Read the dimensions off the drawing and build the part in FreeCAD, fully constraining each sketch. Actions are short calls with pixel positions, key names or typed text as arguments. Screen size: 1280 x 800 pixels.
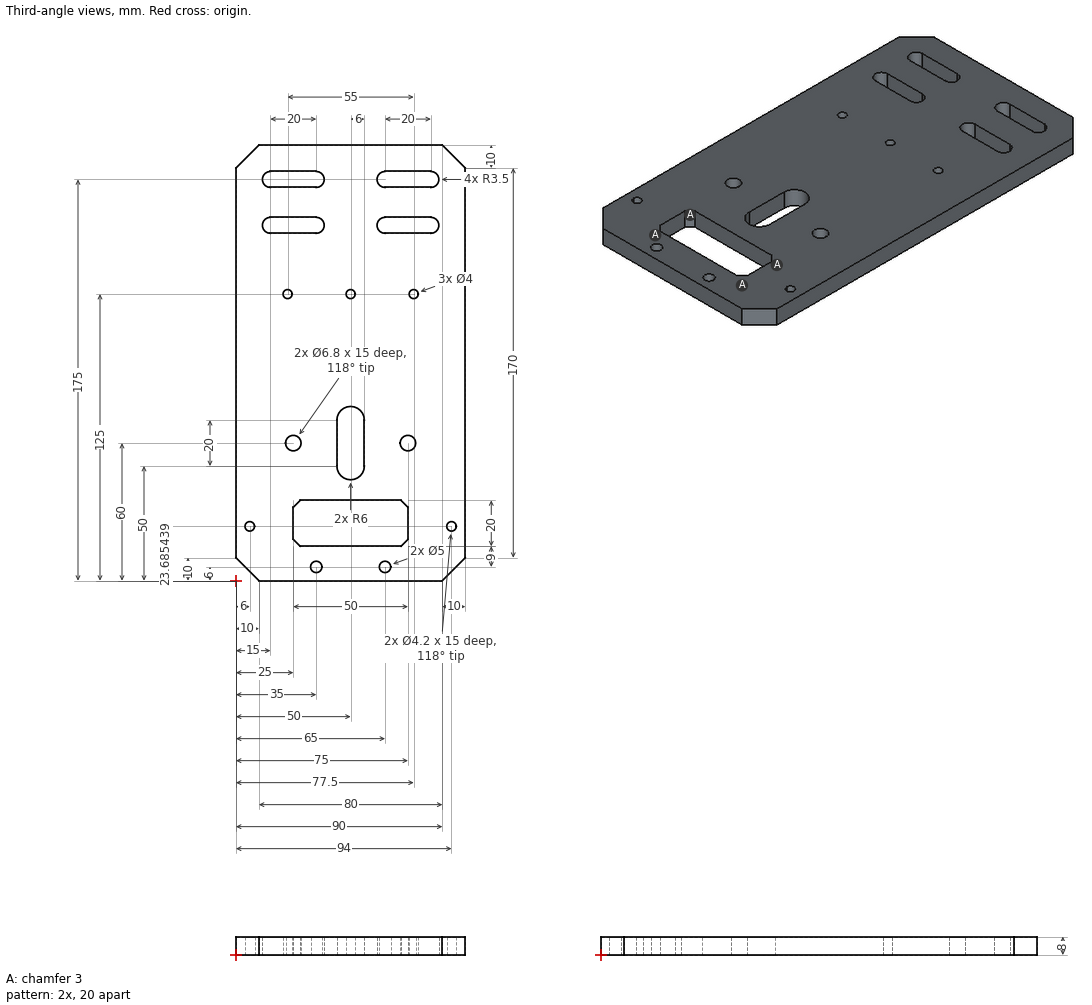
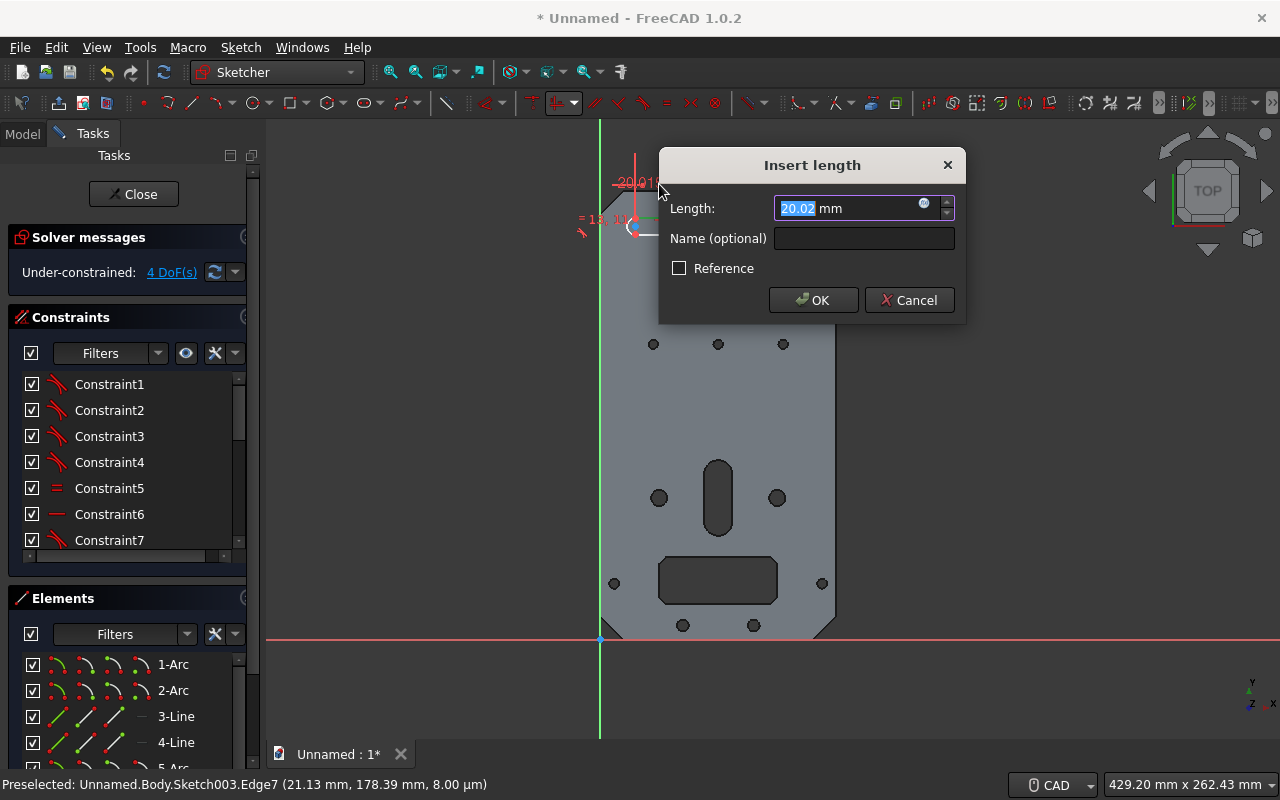
text(20)
key(Return)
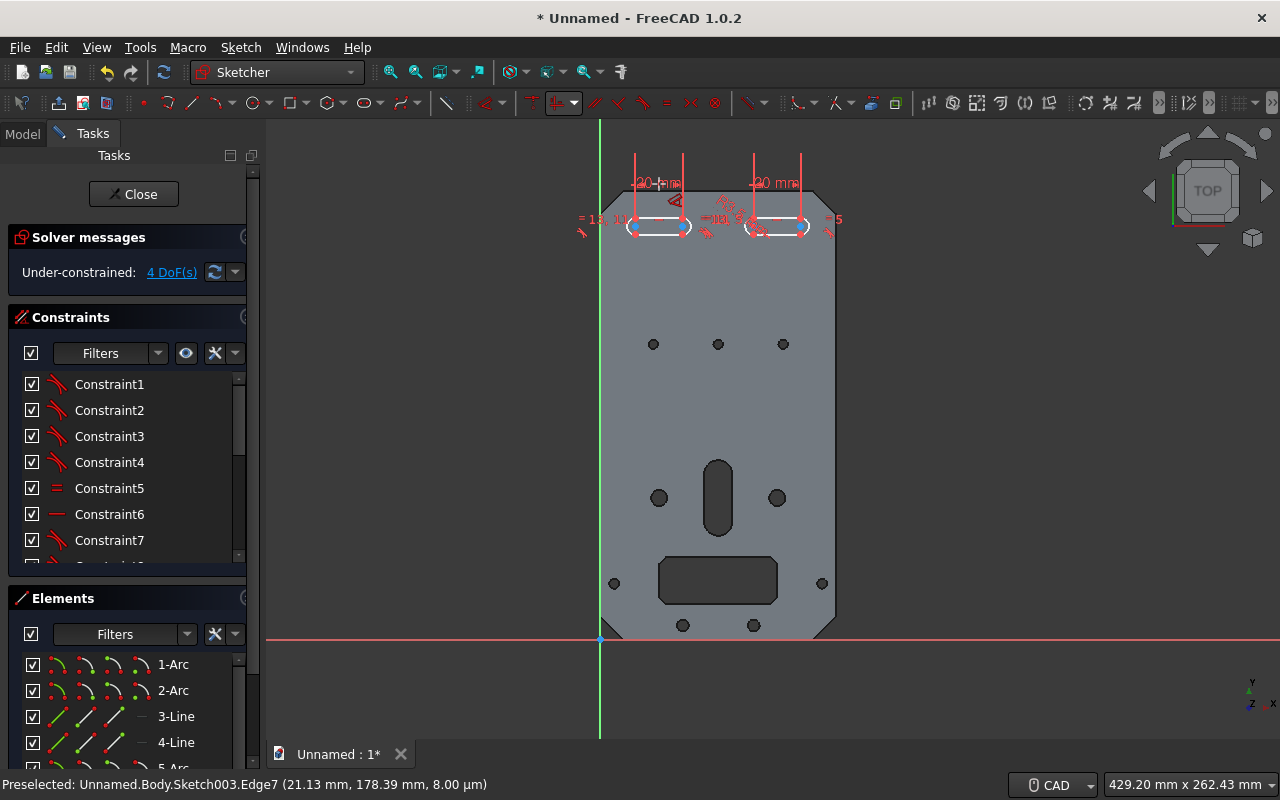
scroll(754, 218, up, 2)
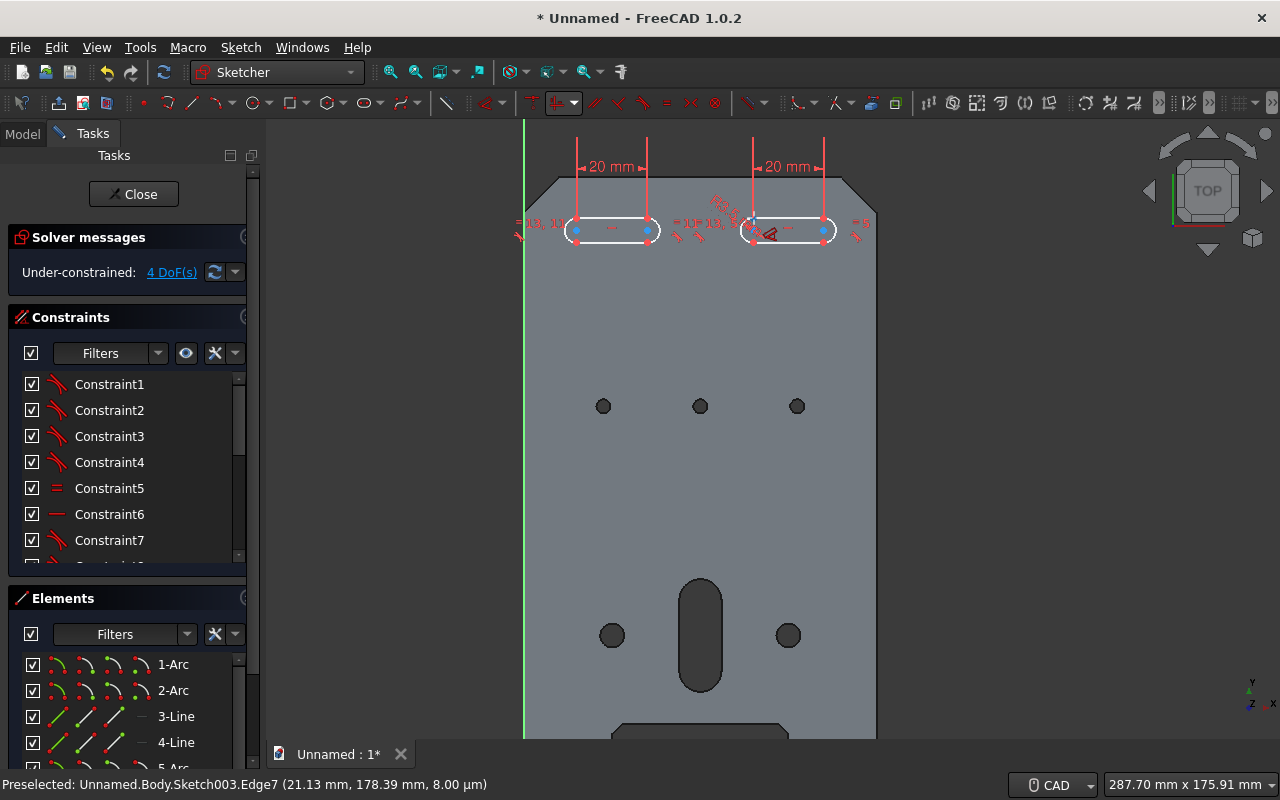
click(753, 218)
click(691, 184)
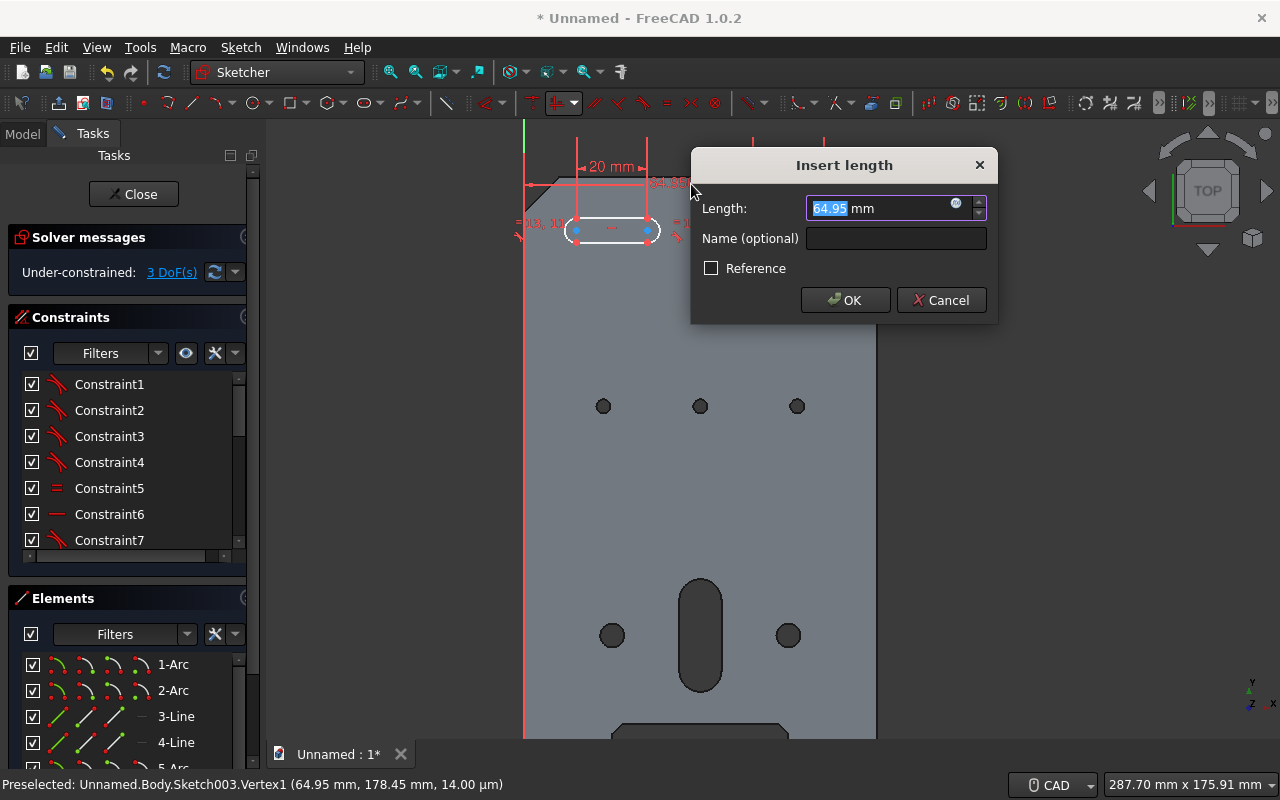
text(65)
key(Return)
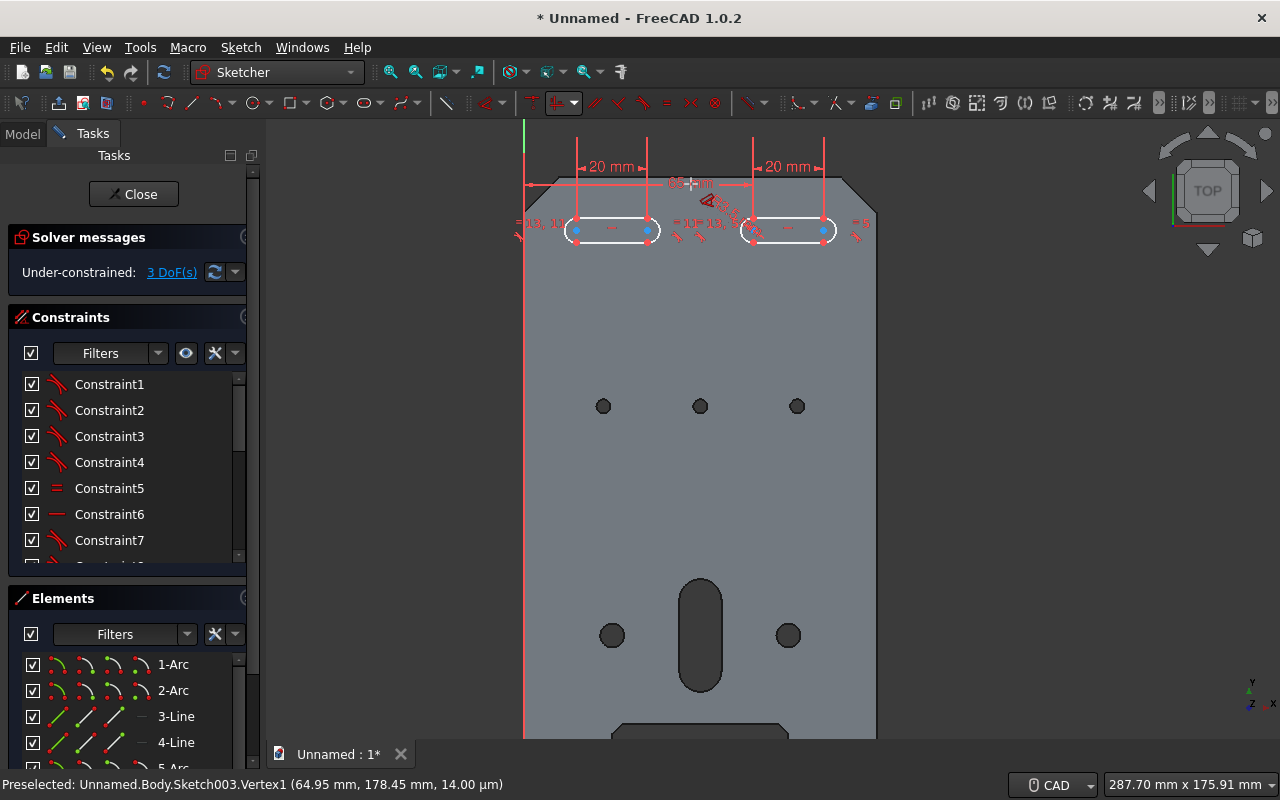
click(577, 218)
click(538, 184)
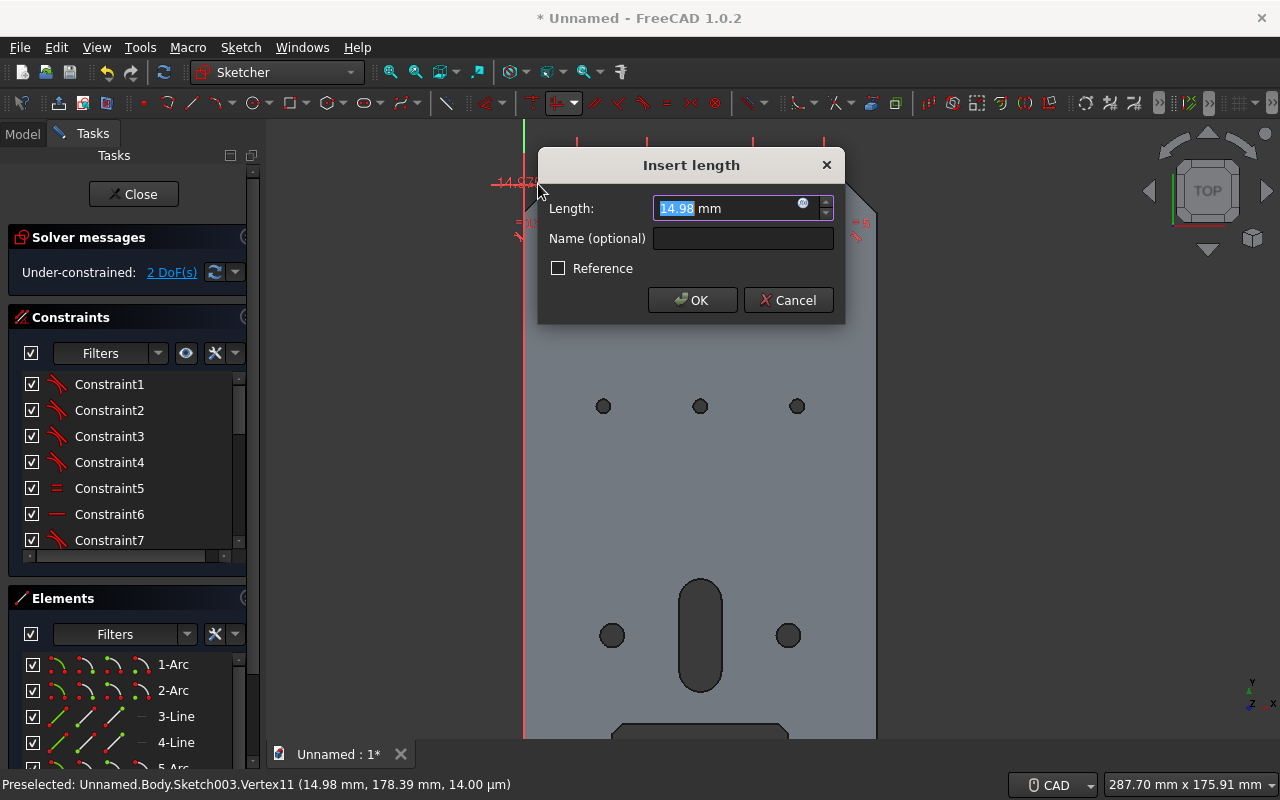
text(15)
key(Return)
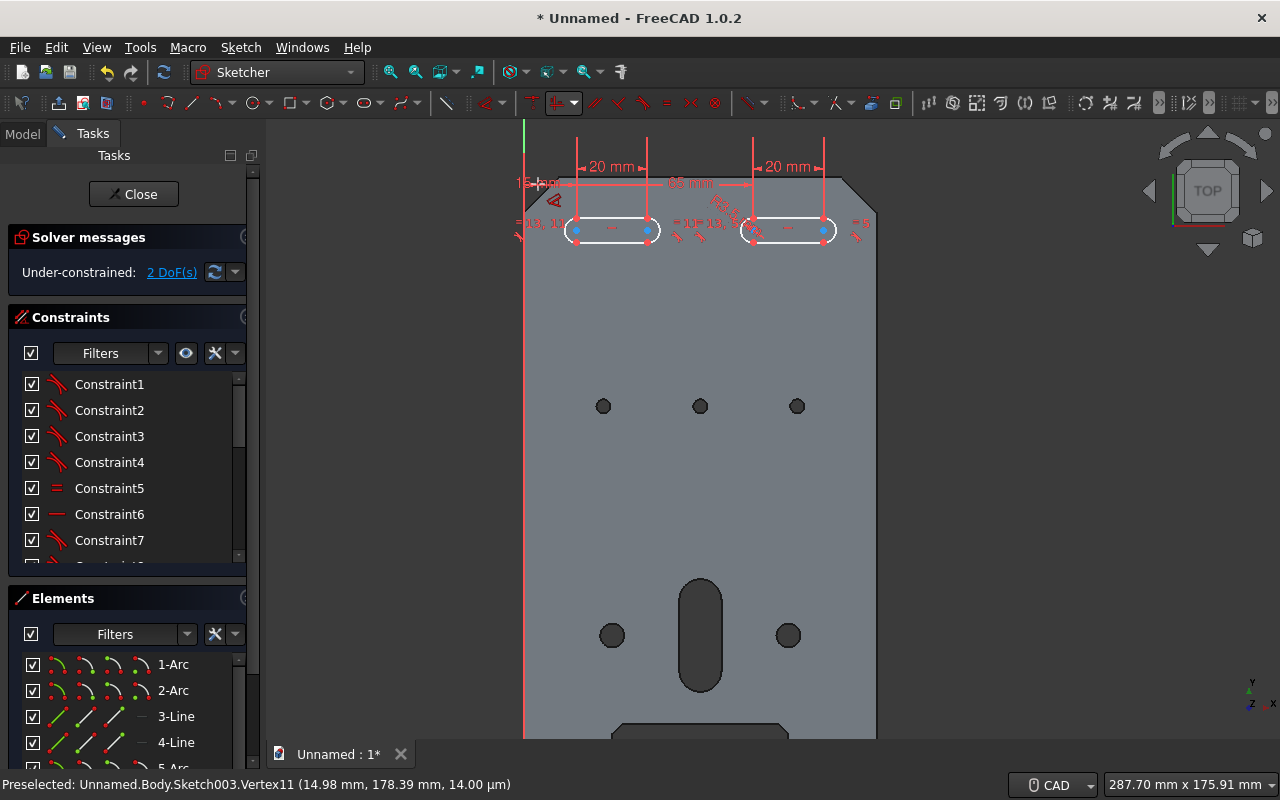
click(753, 230)
click(490, 471)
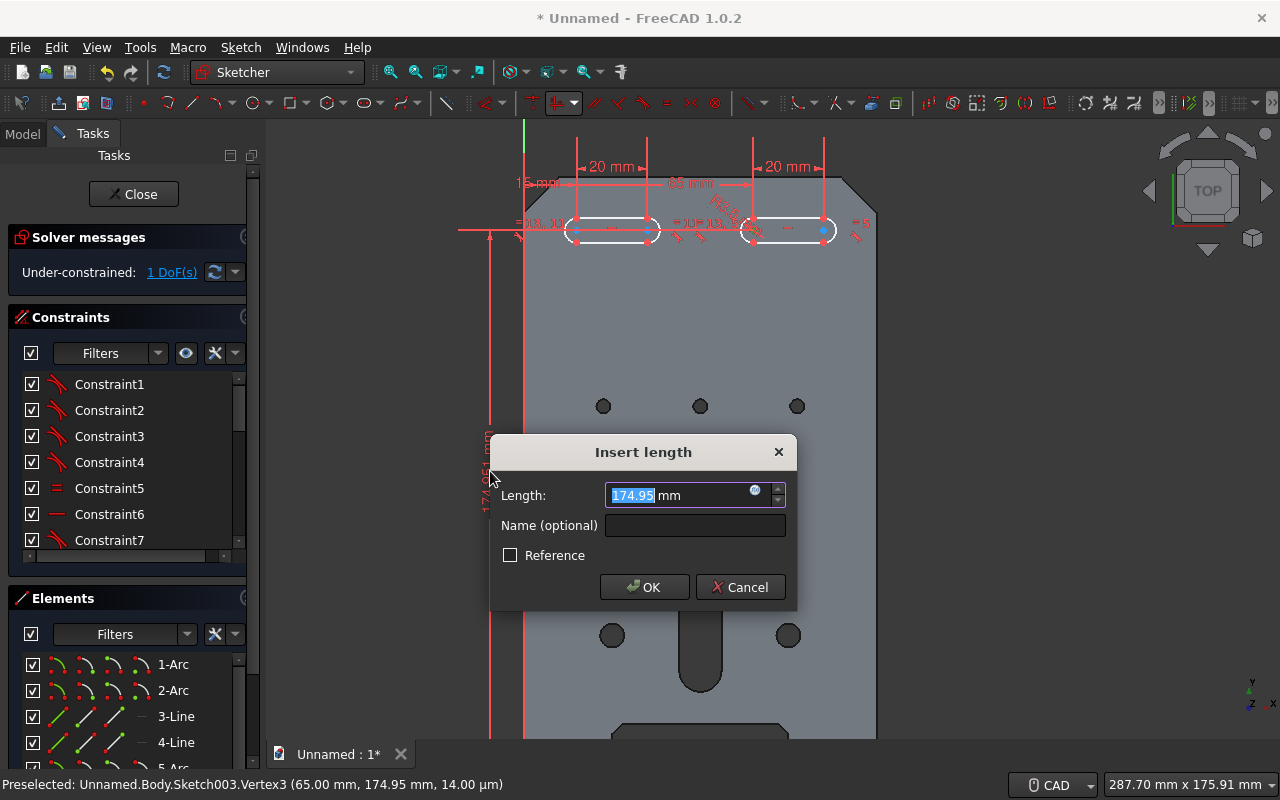
text(175)
key(Return)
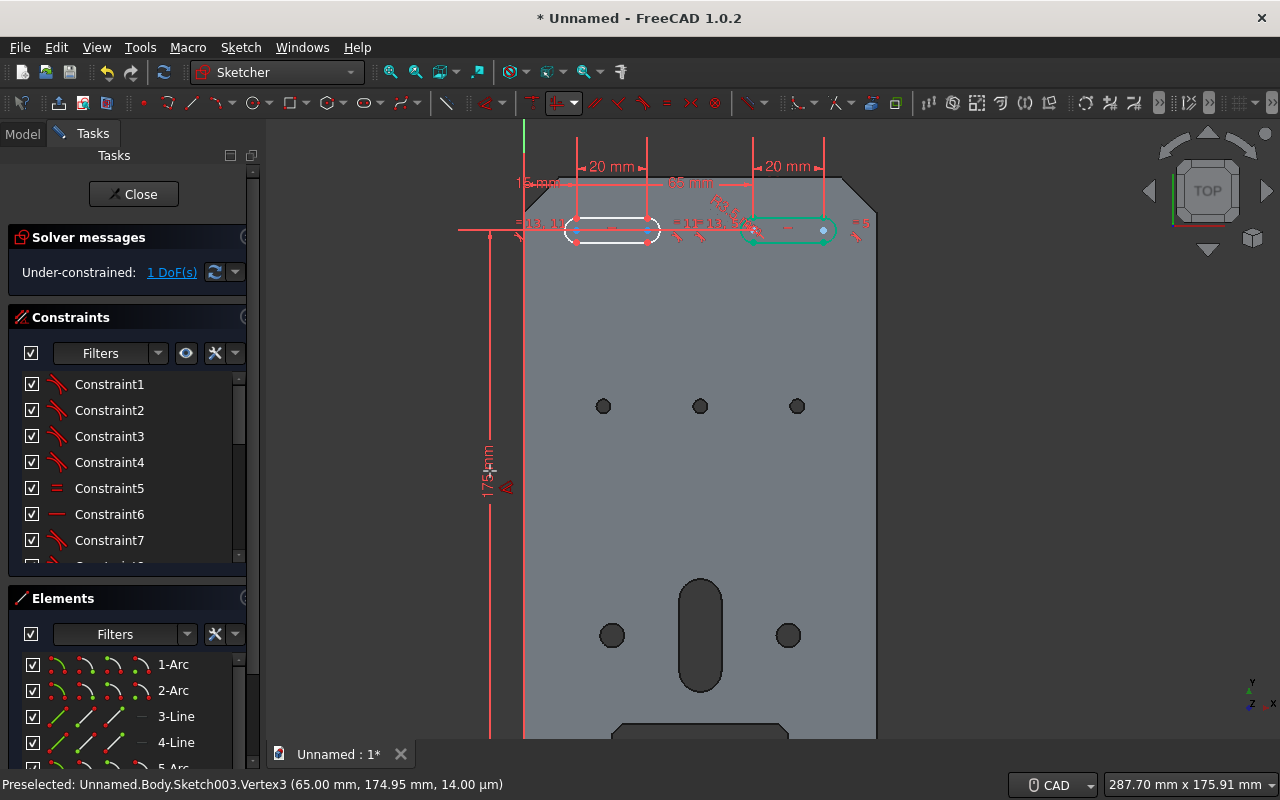
click(577, 231)
click(490, 360)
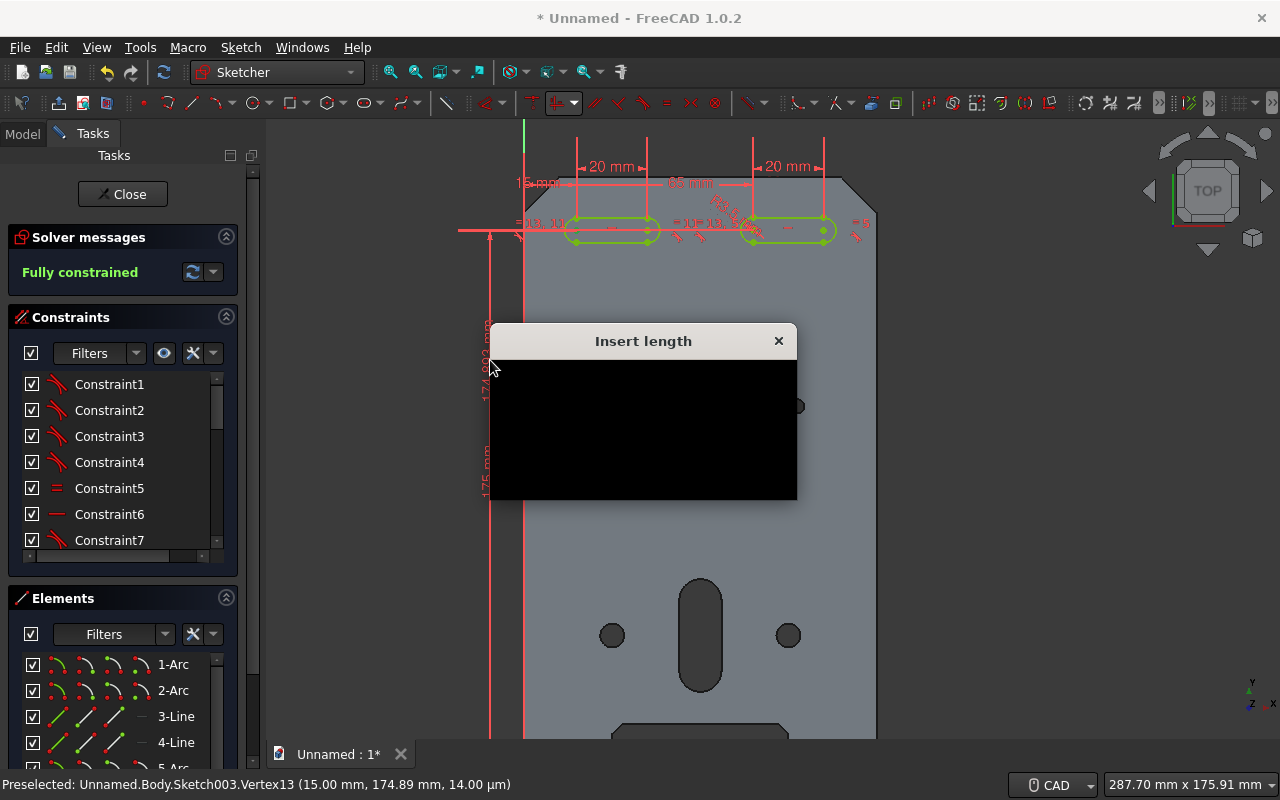
text(175)
key(Return)
key(Escape)